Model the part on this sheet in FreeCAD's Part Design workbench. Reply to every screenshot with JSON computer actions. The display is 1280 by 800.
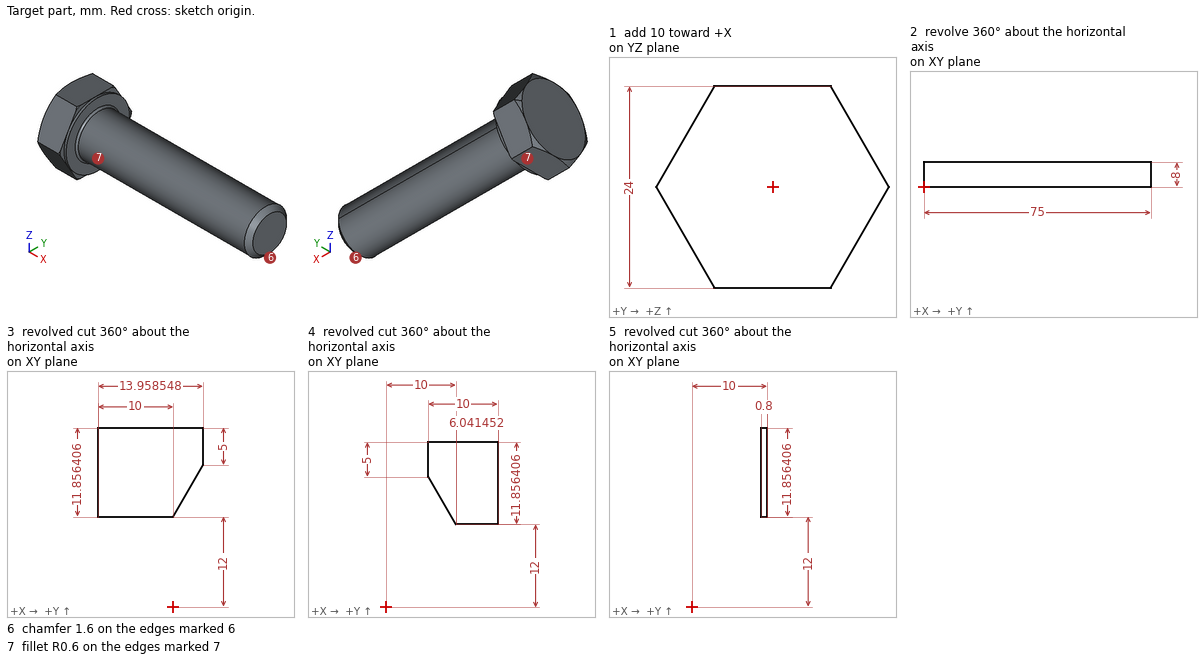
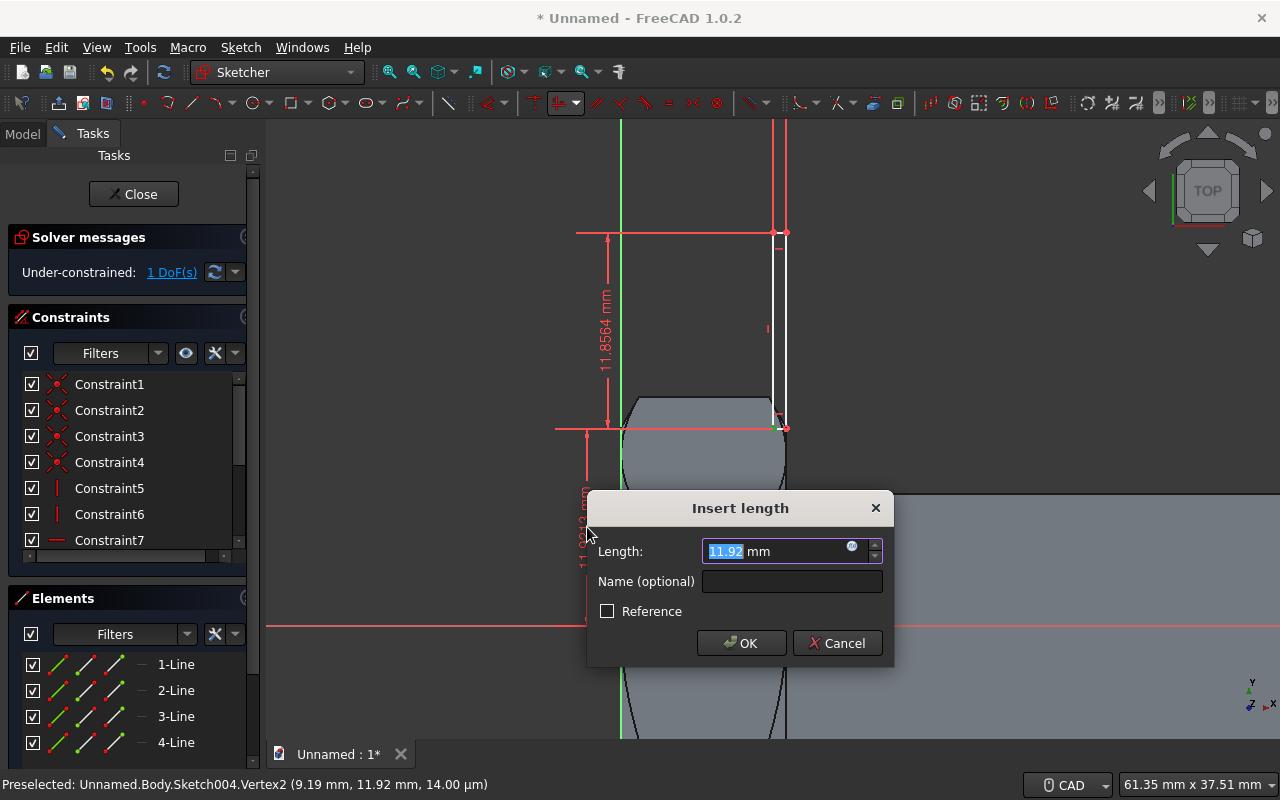
{"action": "type", "text": "12"}
{"action": "key", "text": "Return"}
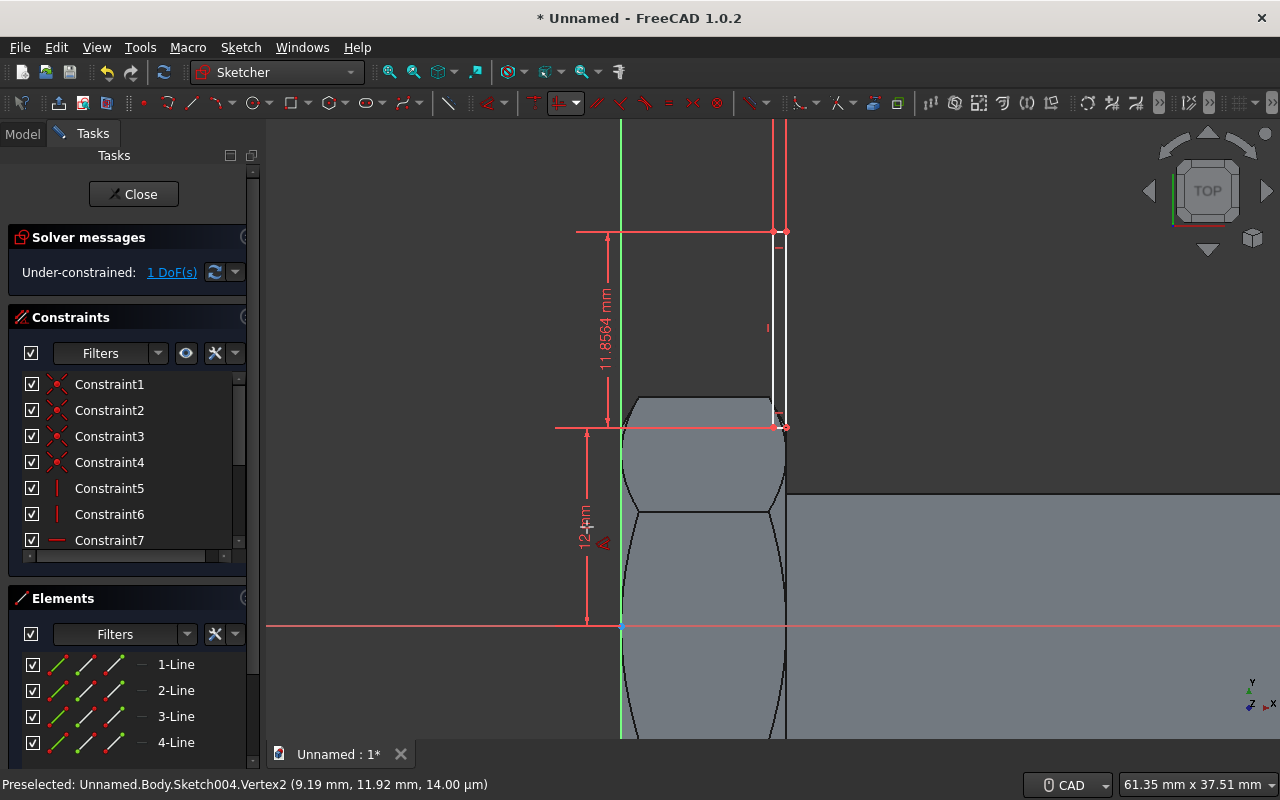
{"action": "left_click", "coordinate": [786, 428]}
{"action": "left_click", "coordinate": [704, 660]}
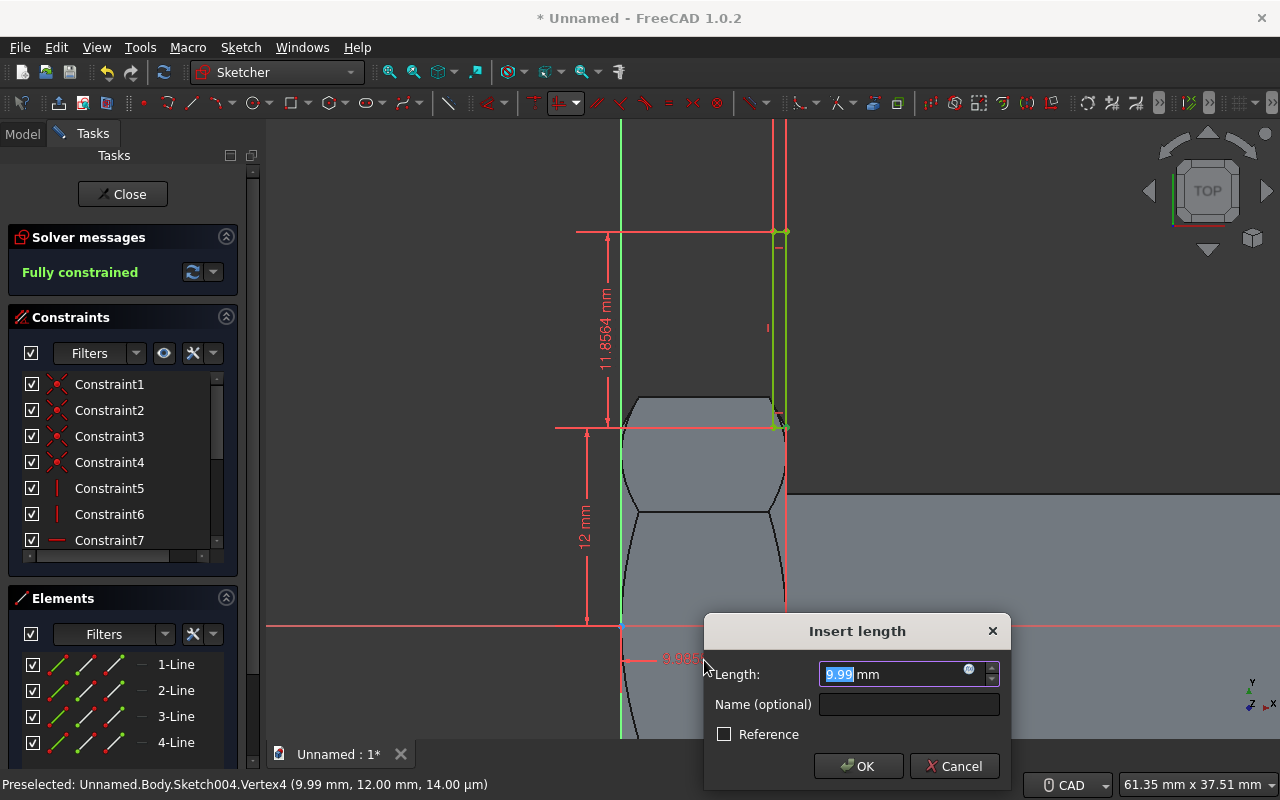
{"action": "type", "text": "10"}
{"action": "key", "text": "Return"}
{"action": "key", "text": "Escape"}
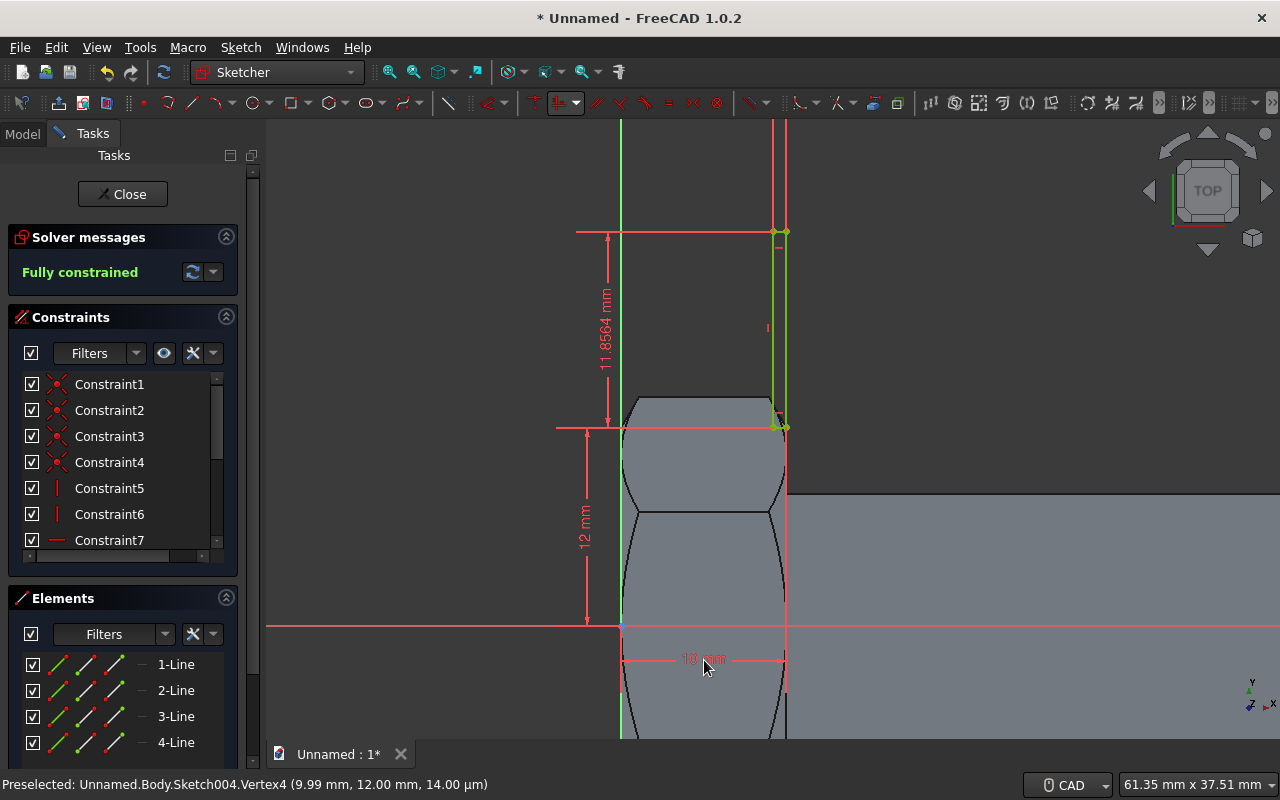
{"action": "left_click", "coordinate": [123, 194]}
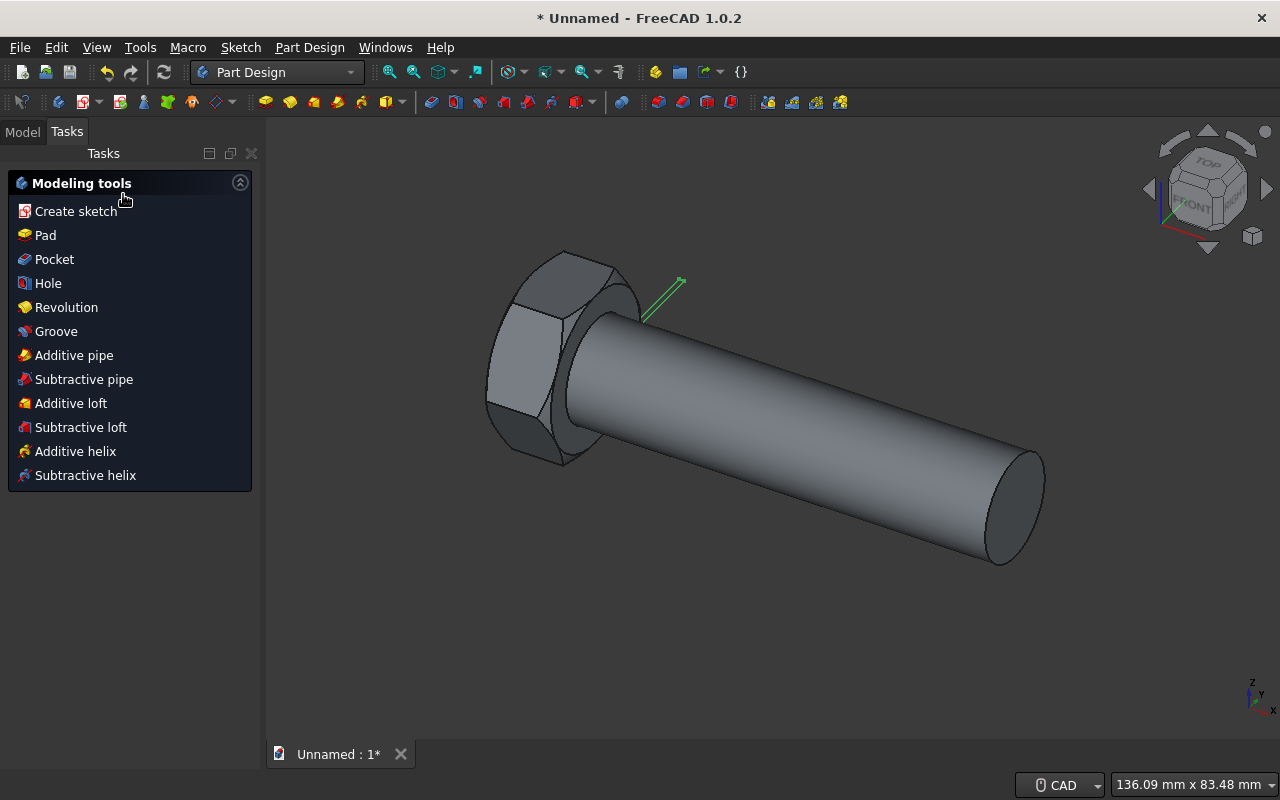
{"action": "left_click", "coordinate": [480, 102]}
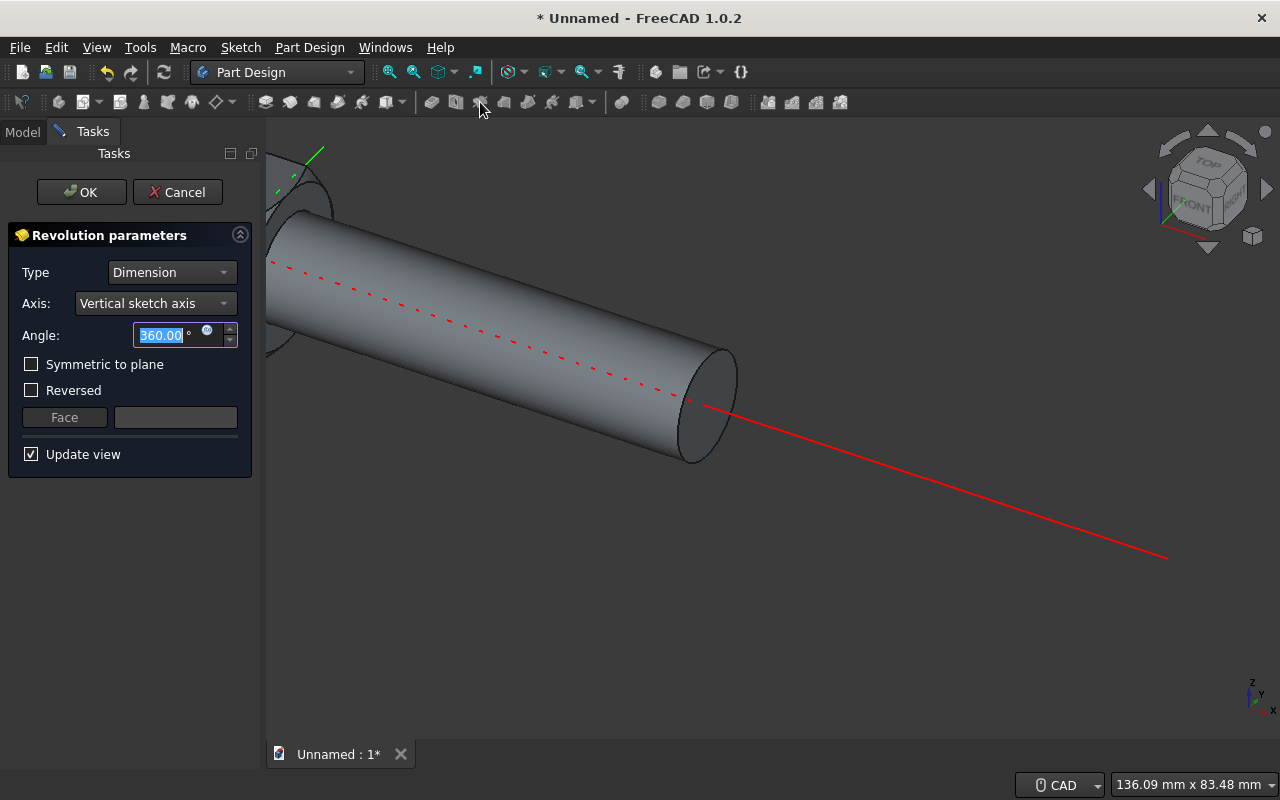
{"action": "left_click", "coordinate": [156, 304]}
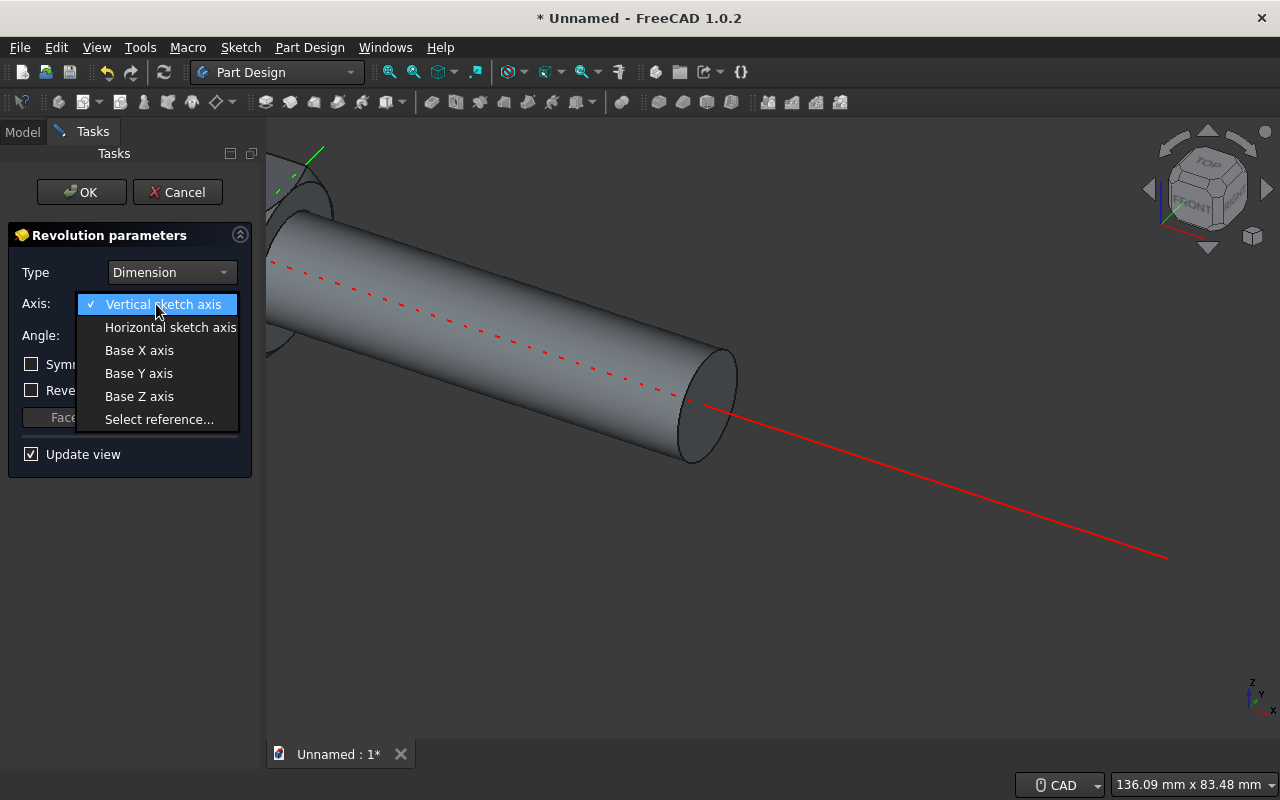
{"action": "left_click", "coordinate": [156, 328]}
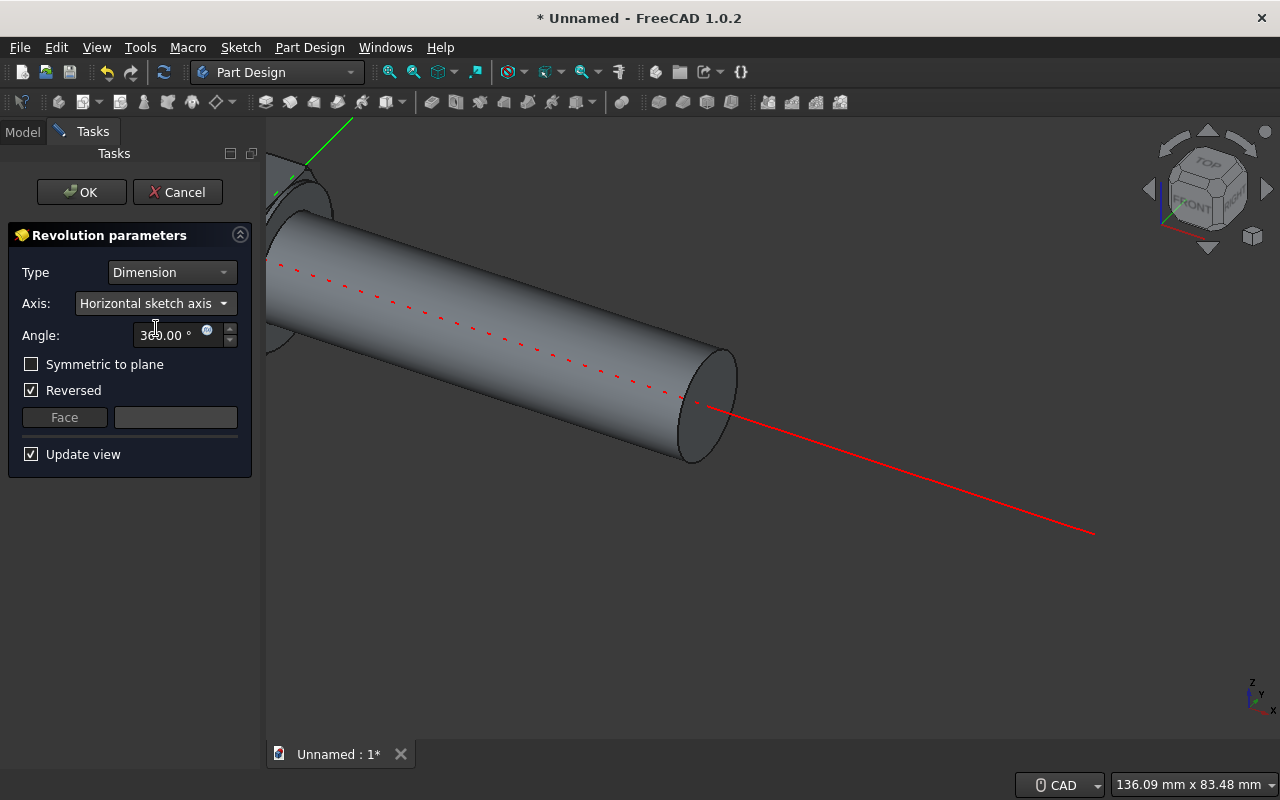
{"action": "left_click", "coordinate": [82, 192]}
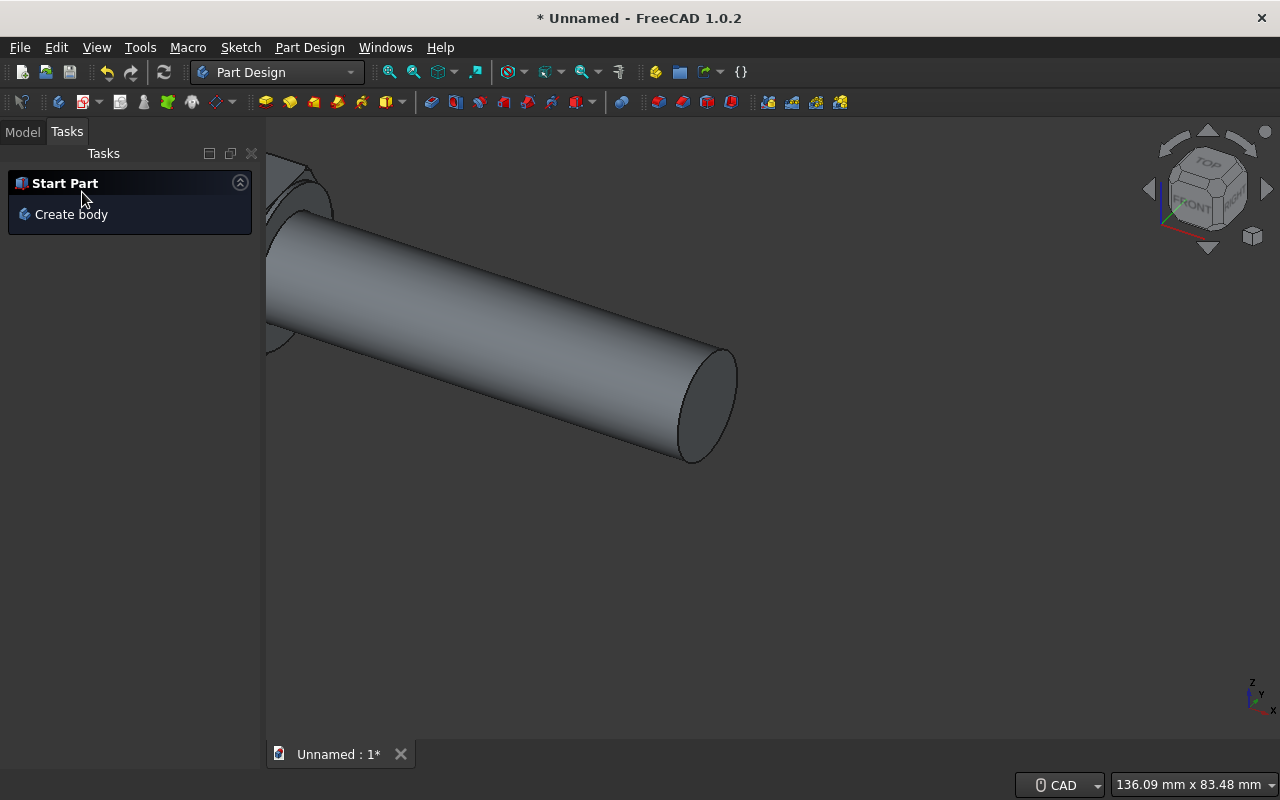
{"action": "left_click", "coordinate": [390, 72]}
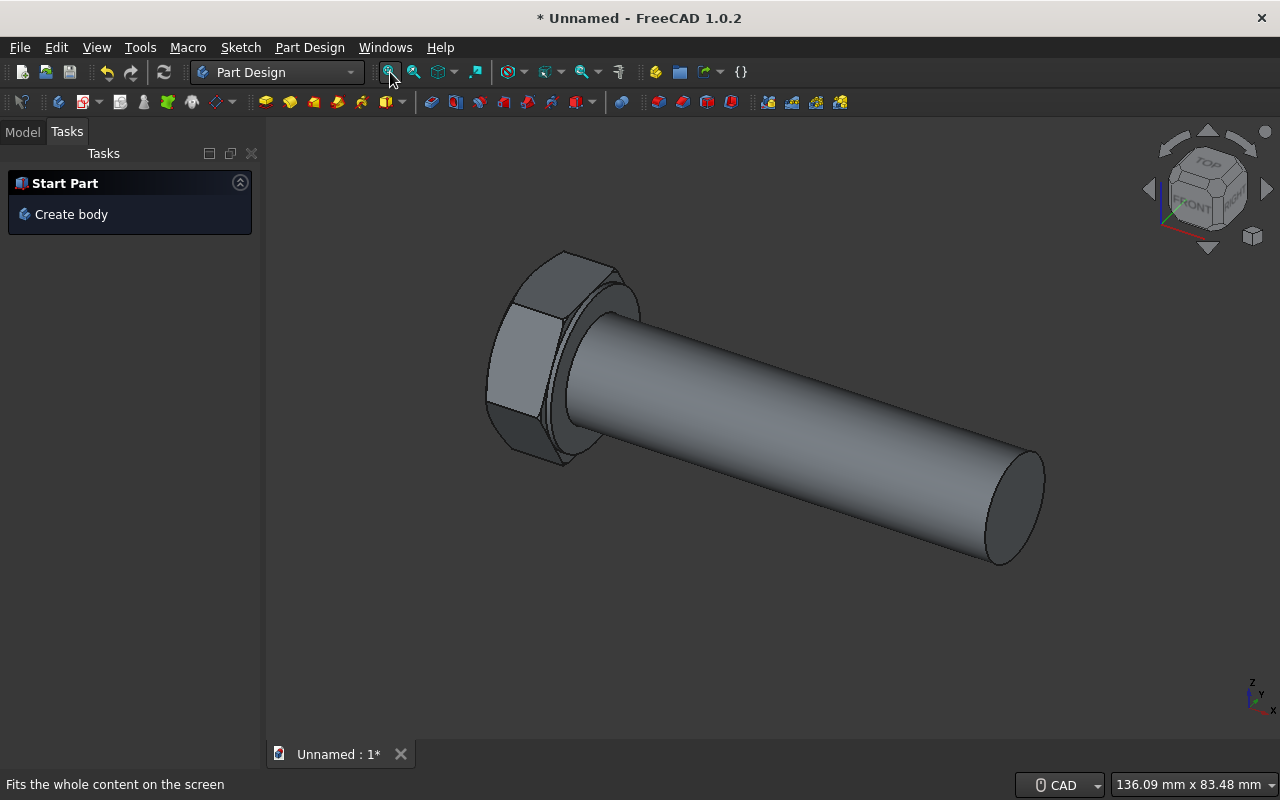
{"action": "left_click", "coordinate": [985, 537]}